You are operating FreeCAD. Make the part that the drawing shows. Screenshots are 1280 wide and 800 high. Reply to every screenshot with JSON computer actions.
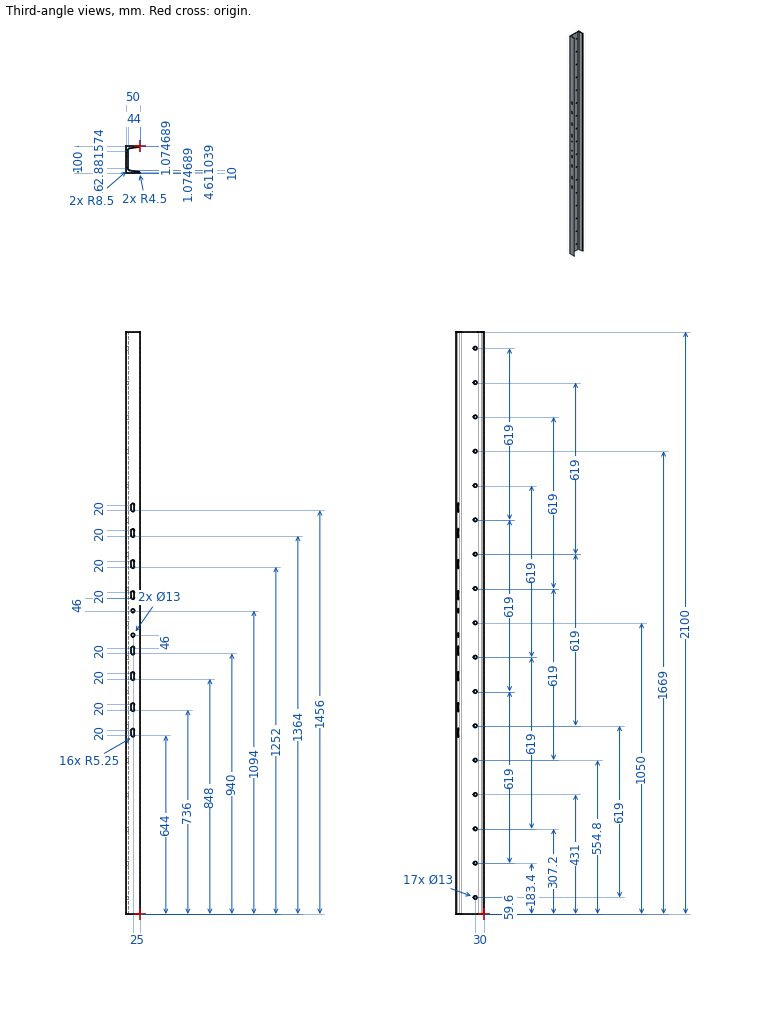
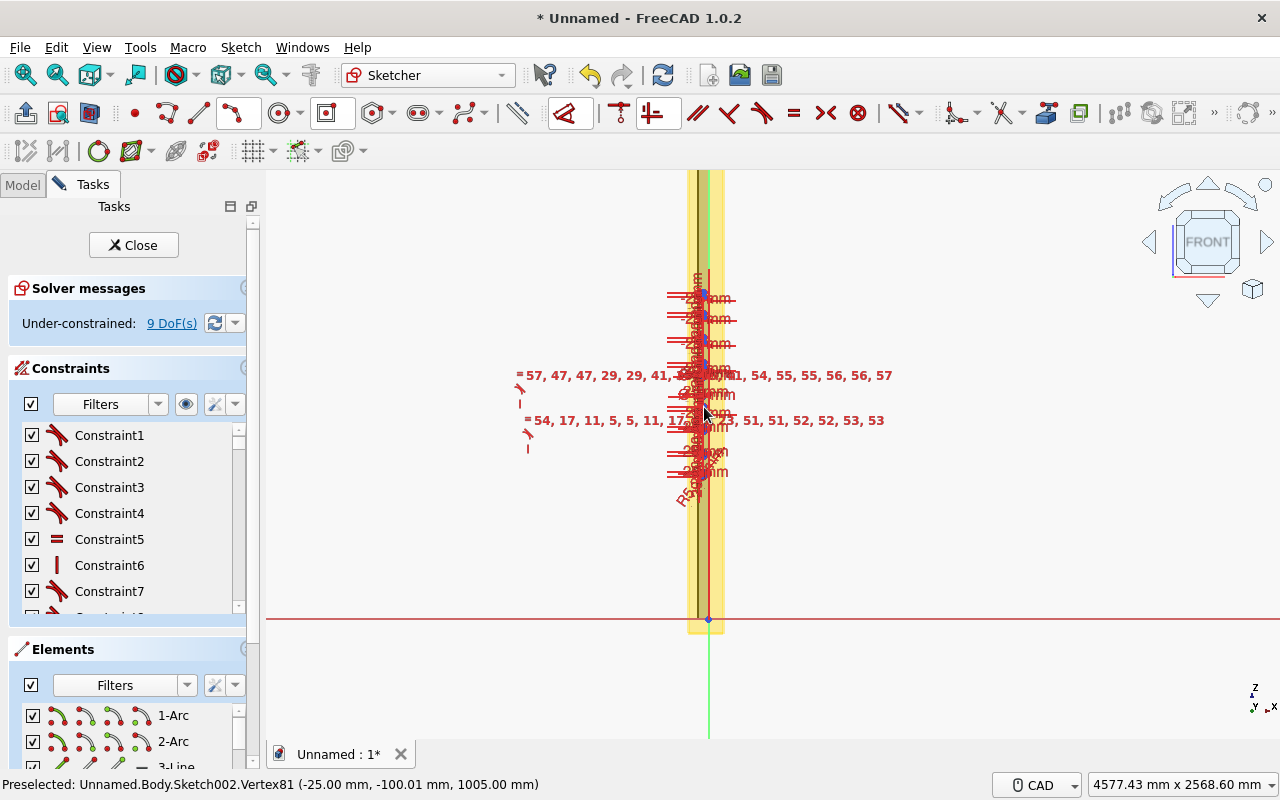
{"action": "scroll", "coordinate": [702, 367], "scroll_direction": "up", "scroll_amount": 12}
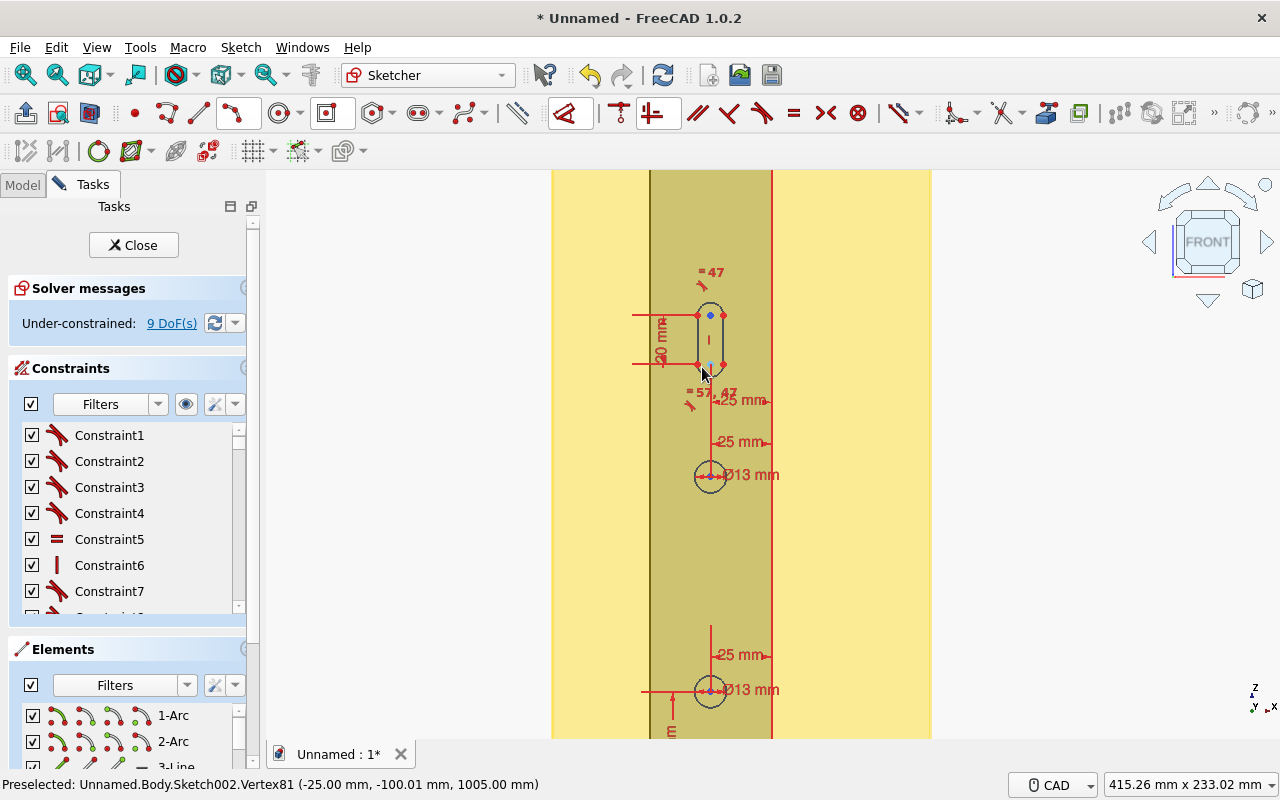
{"action": "left_click", "coordinate": [698, 364]}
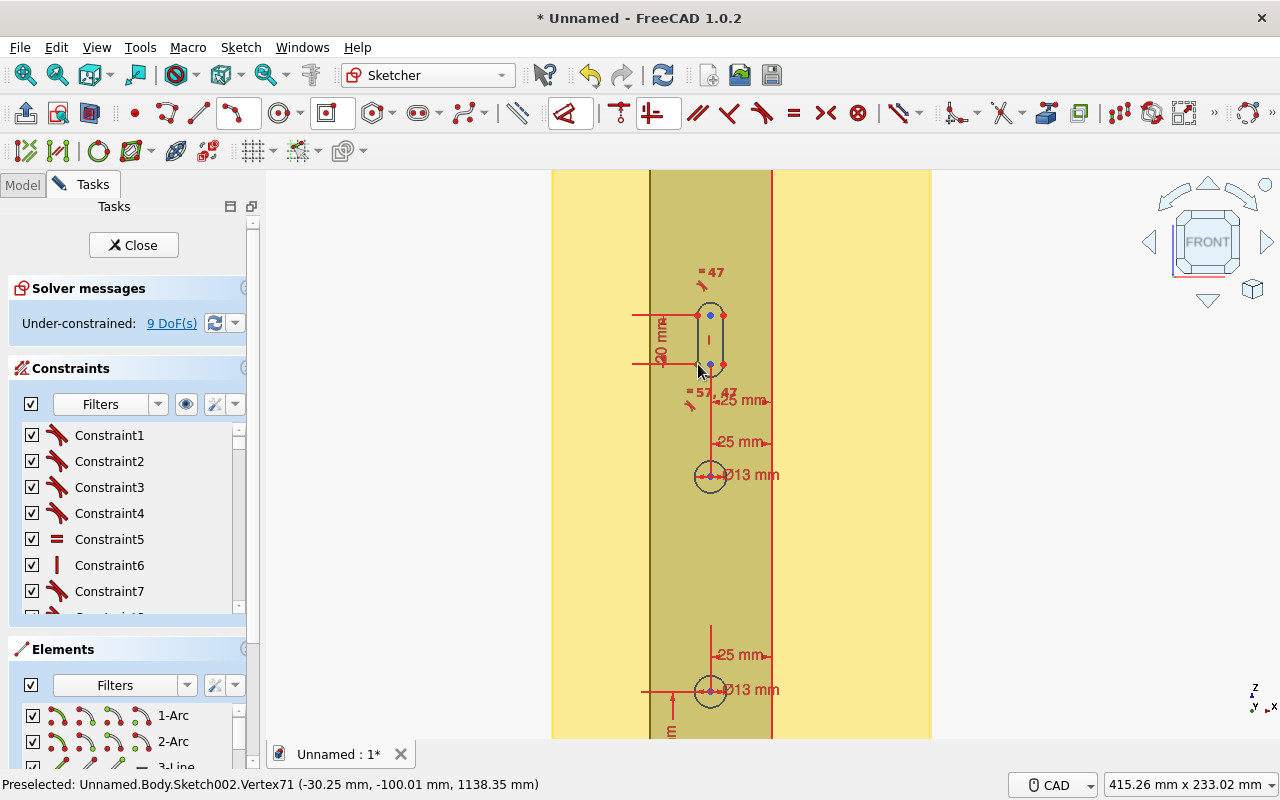
{"action": "left_click", "coordinate": [711, 477]}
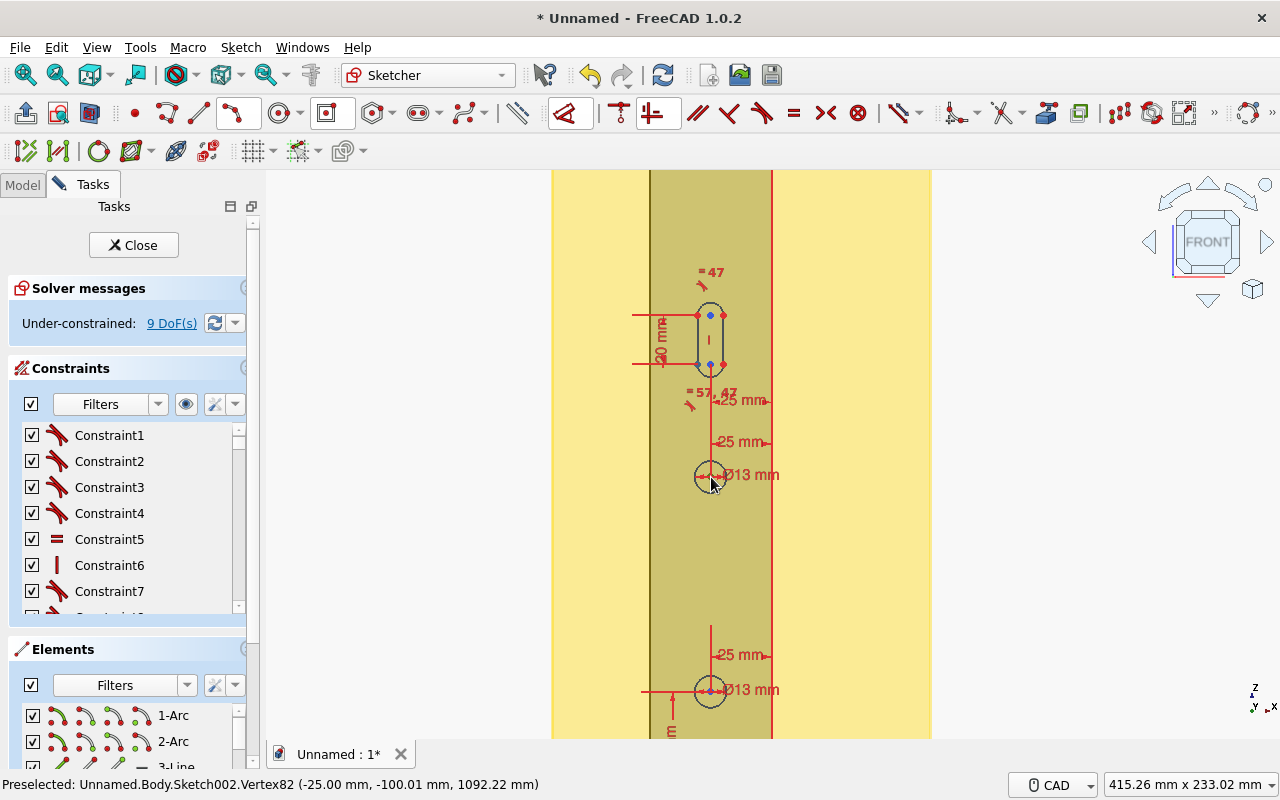
{"action": "left_click", "coordinate": [588, 114]}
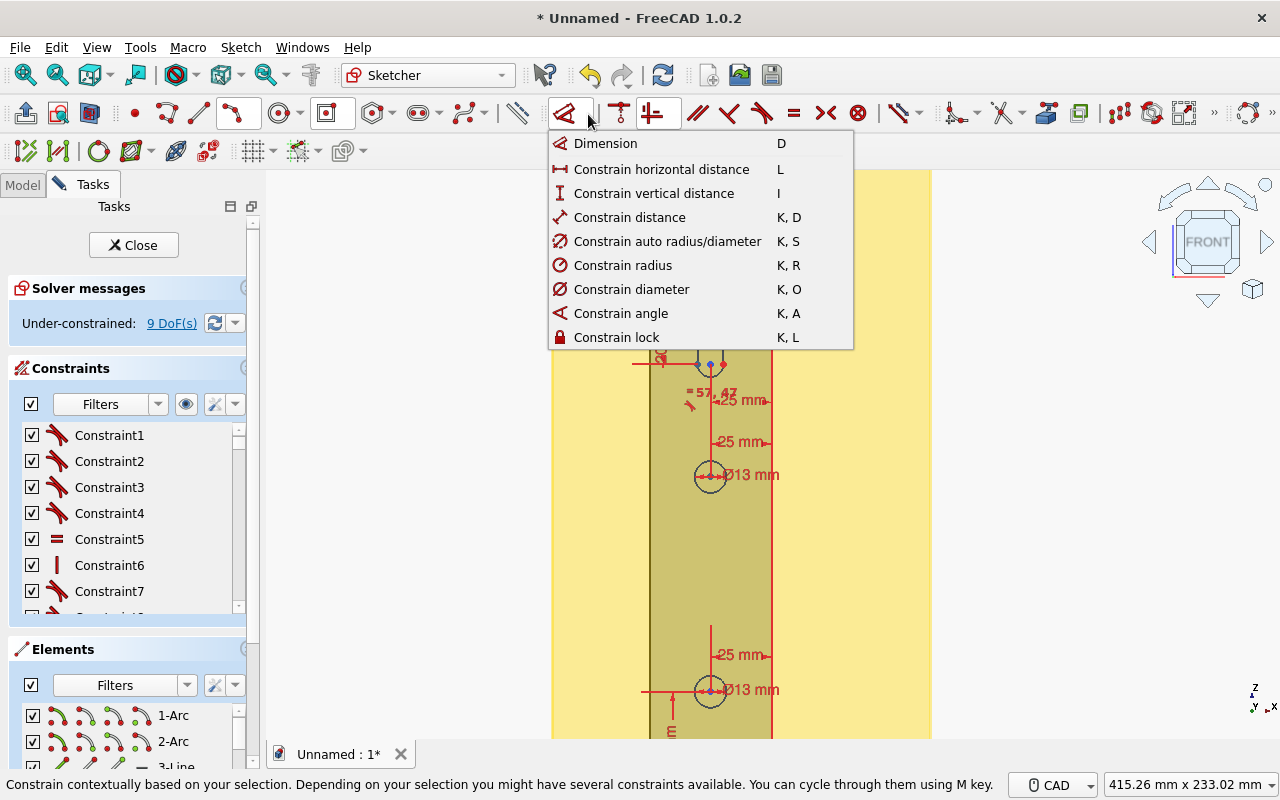
{"action": "left_click", "coordinate": [701, 193]}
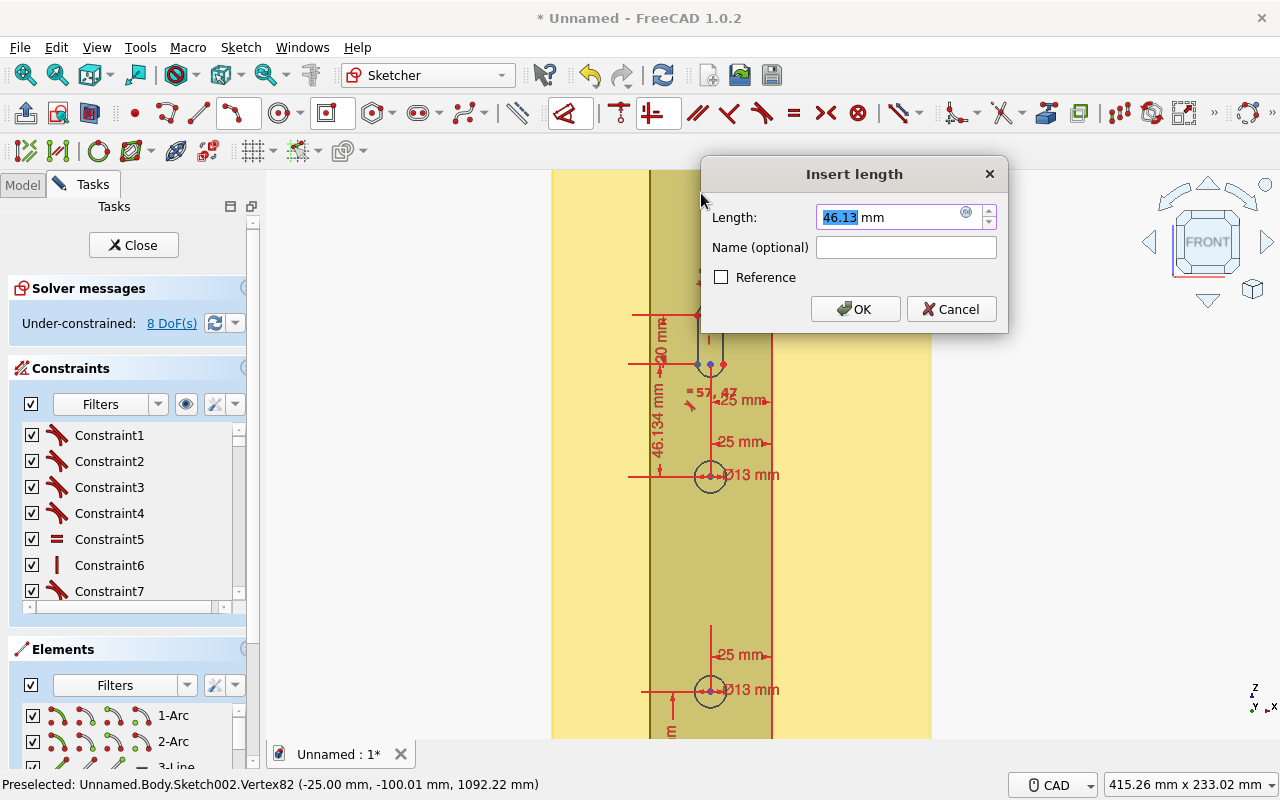
{"action": "type", "text": "46"}
{"action": "key", "text": "Return"}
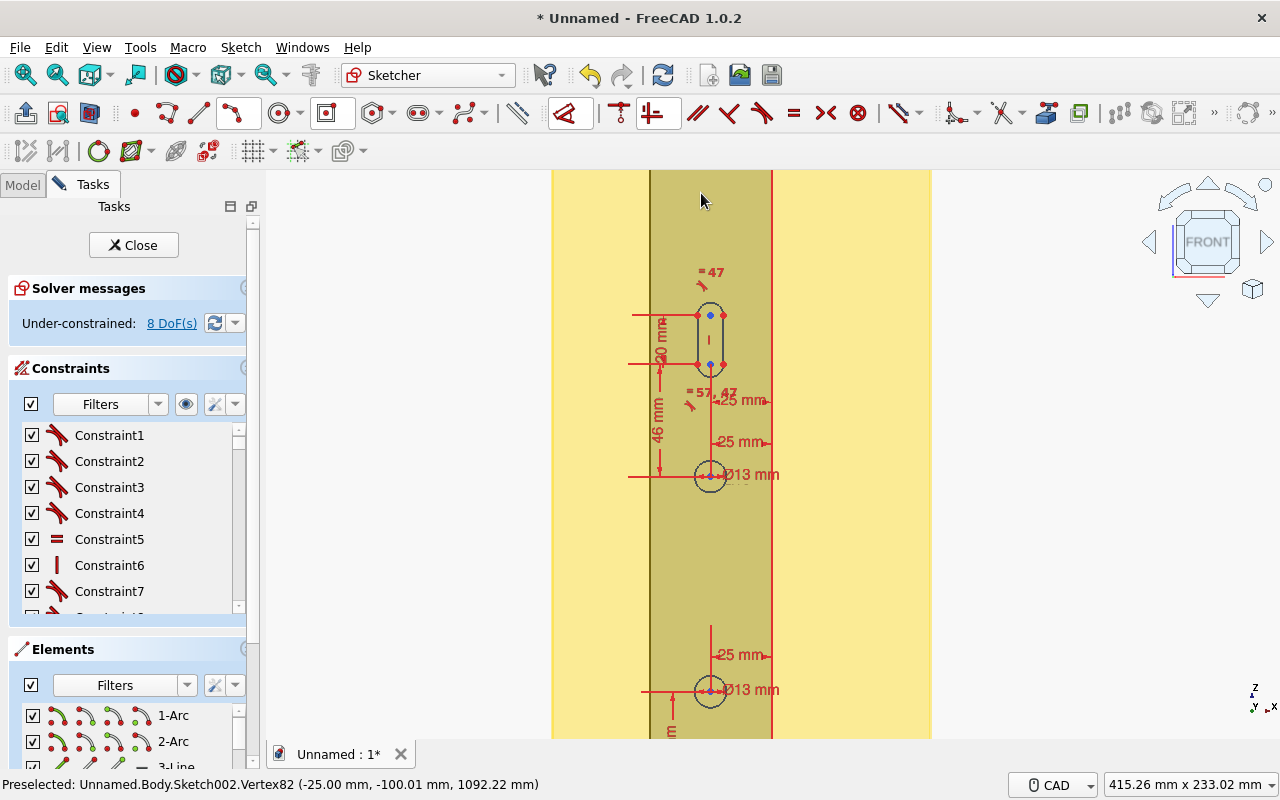
{"action": "scroll", "coordinate": [702, 367], "scroll_direction": "down", "scroll_amount": 12}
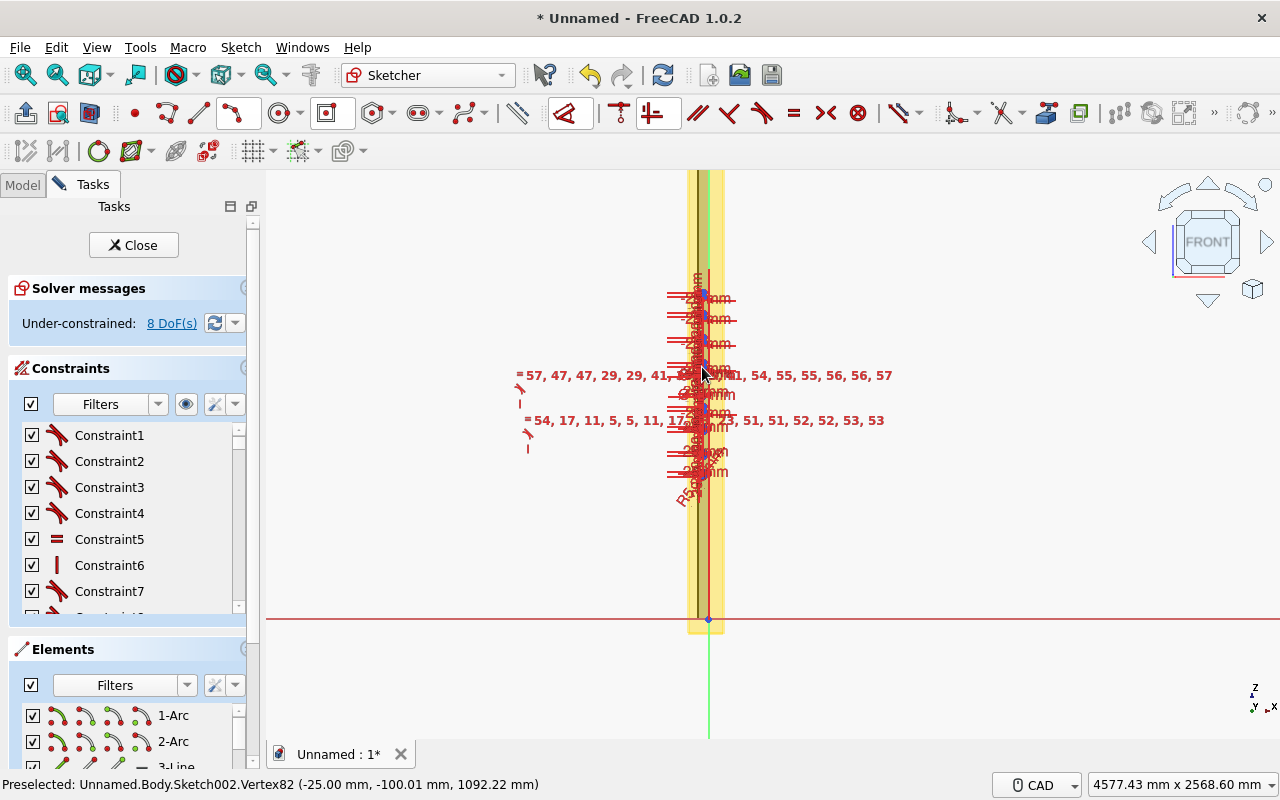
{"action": "scroll", "coordinate": [702, 477], "scroll_direction": "up", "scroll_amount": 12}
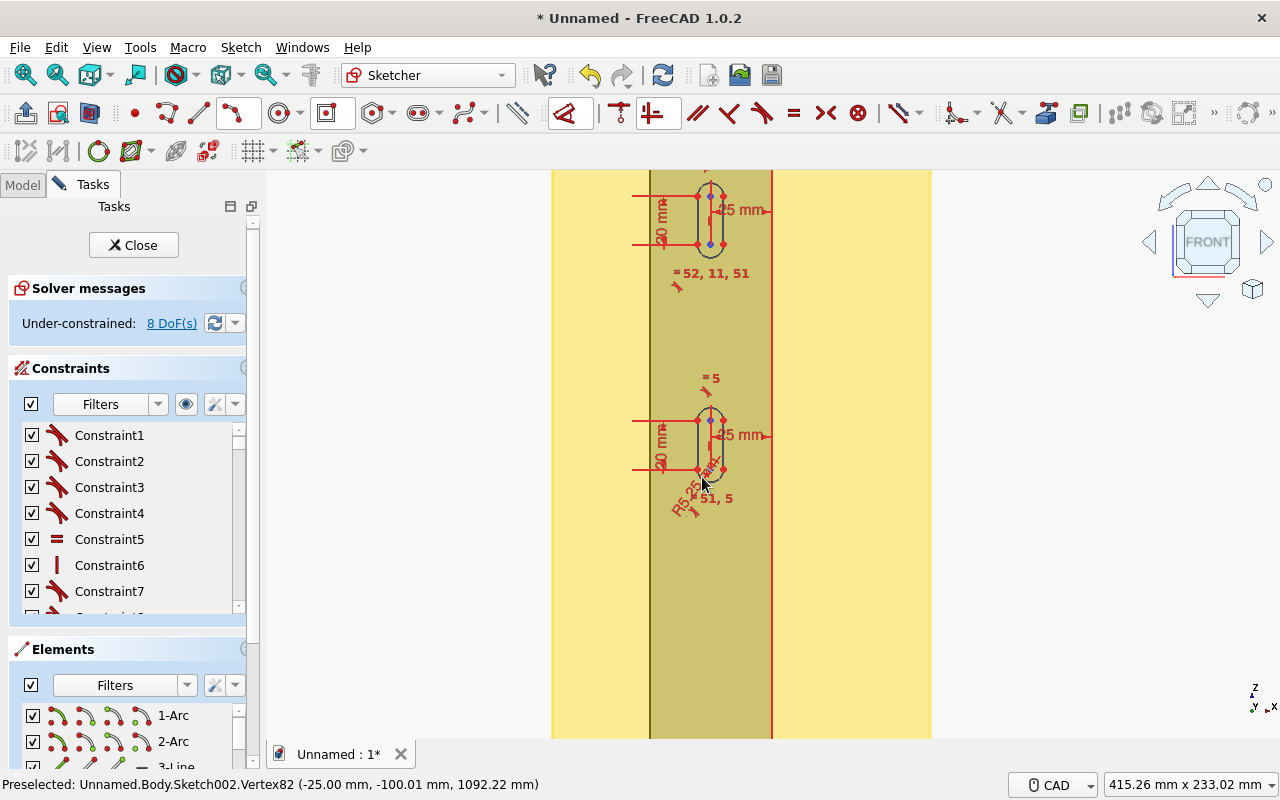
{"action": "left_click", "coordinate": [698, 470]}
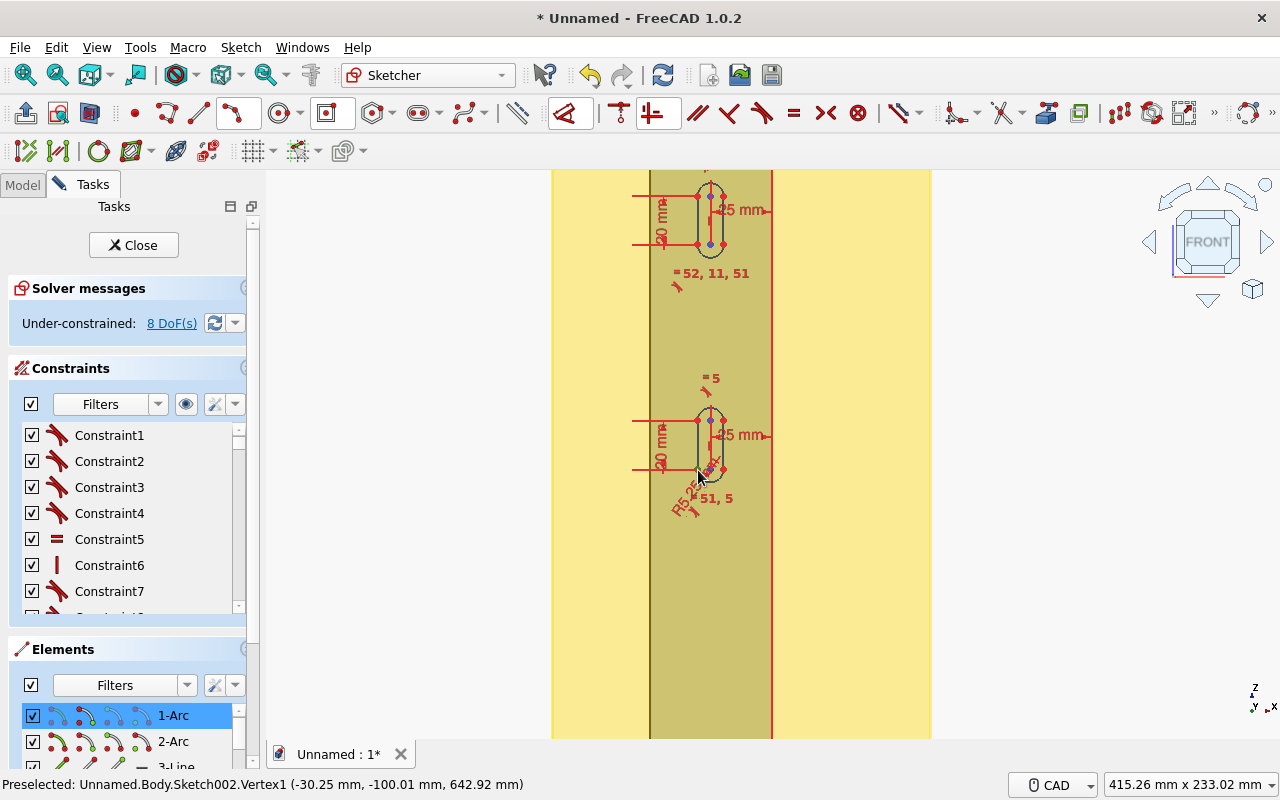
{"action": "key", "text": "i"}